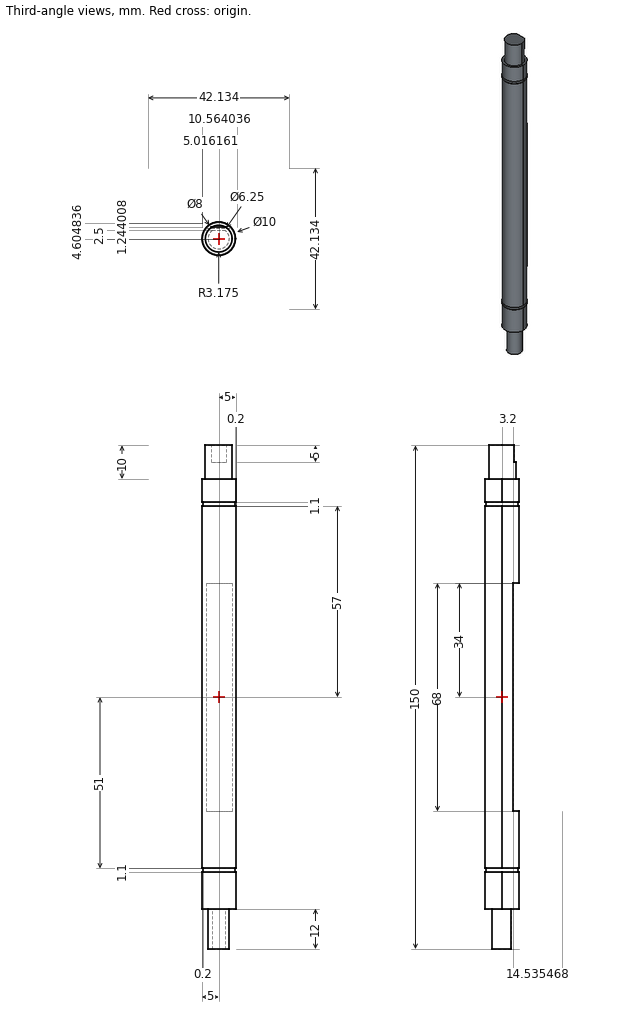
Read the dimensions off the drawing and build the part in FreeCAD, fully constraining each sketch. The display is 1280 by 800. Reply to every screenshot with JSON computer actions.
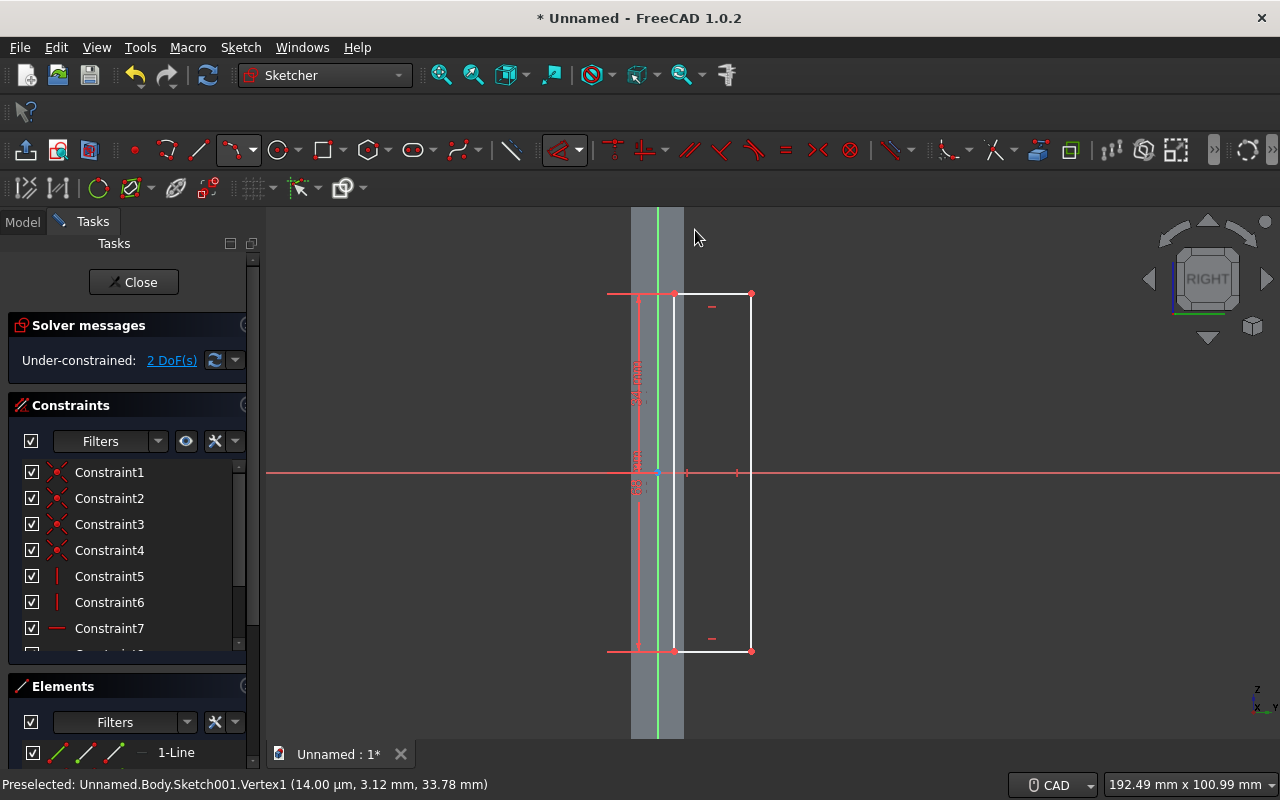
{"action": "scroll", "coordinate": [674, 294], "scroll_direction": "up", "scroll_amount": 5}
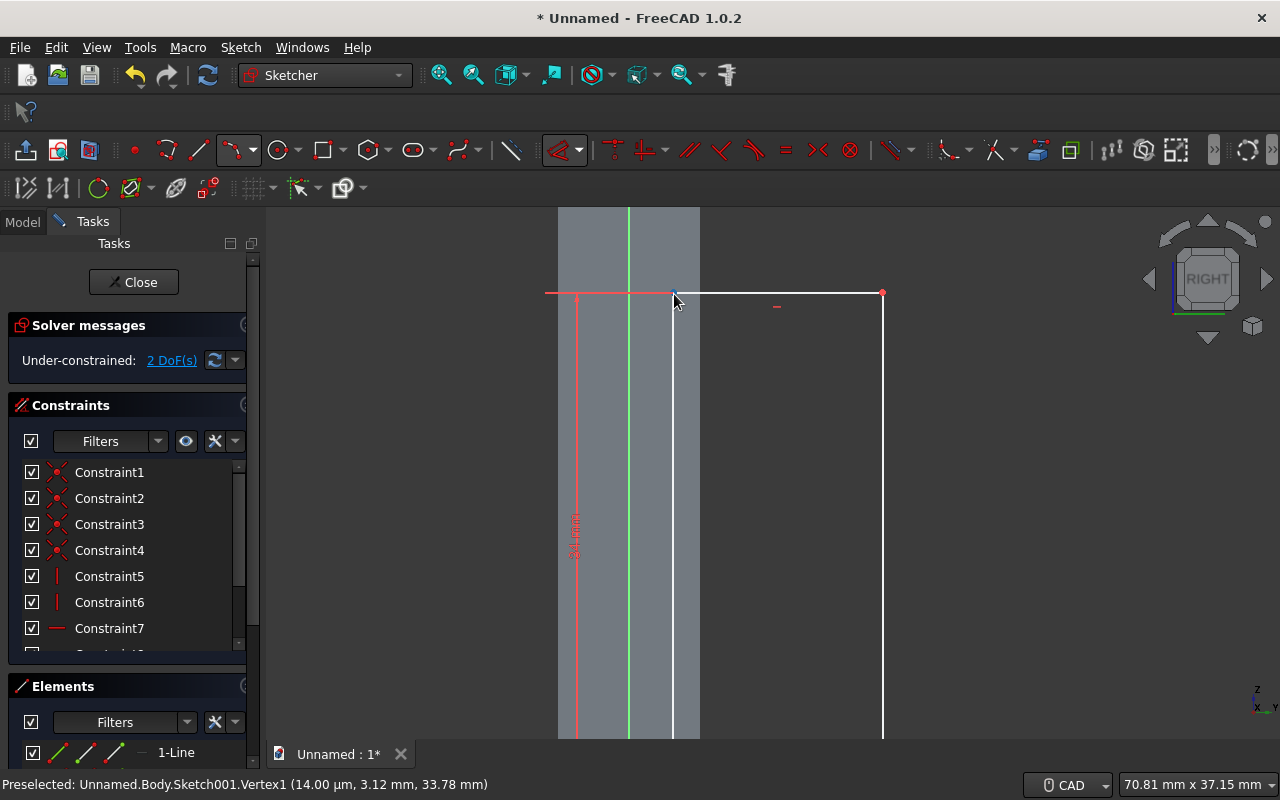
{"action": "left_click", "coordinate": [673, 293]}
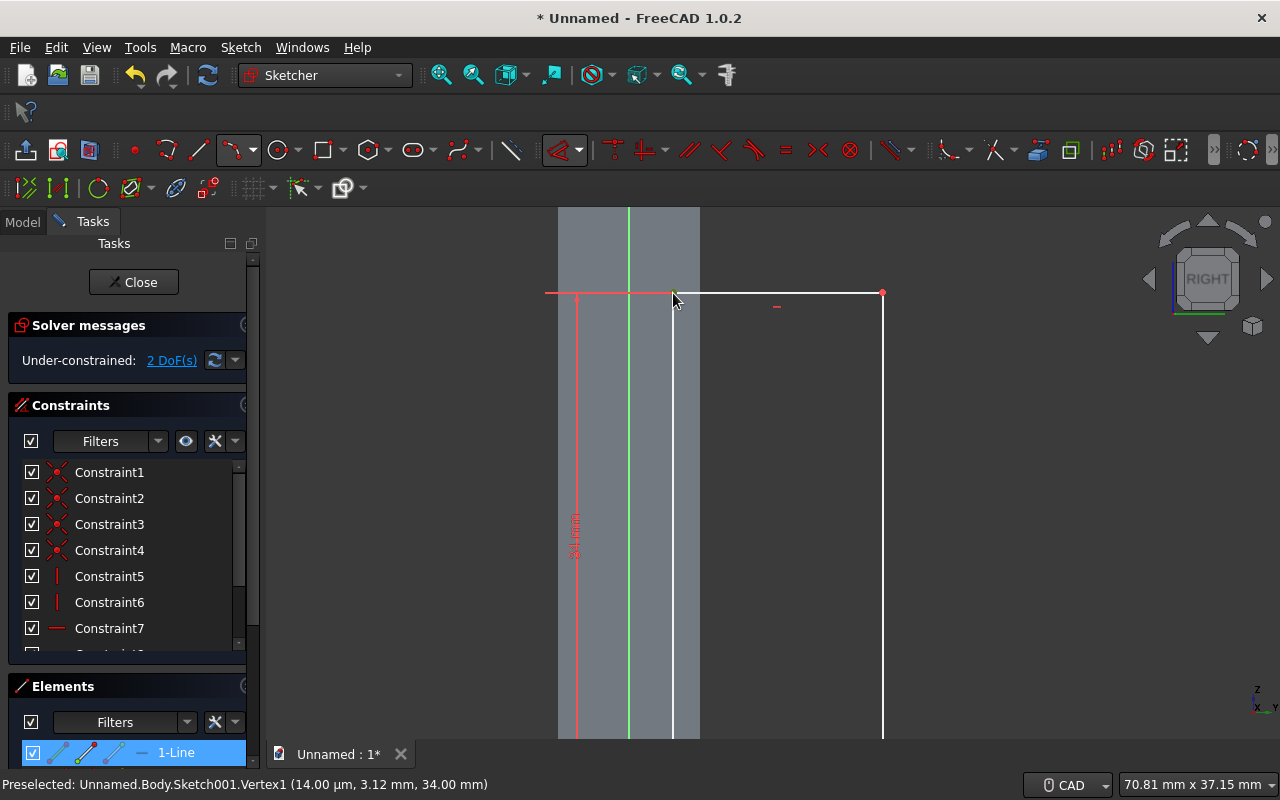
{"action": "left_click", "coordinate": [582, 150]}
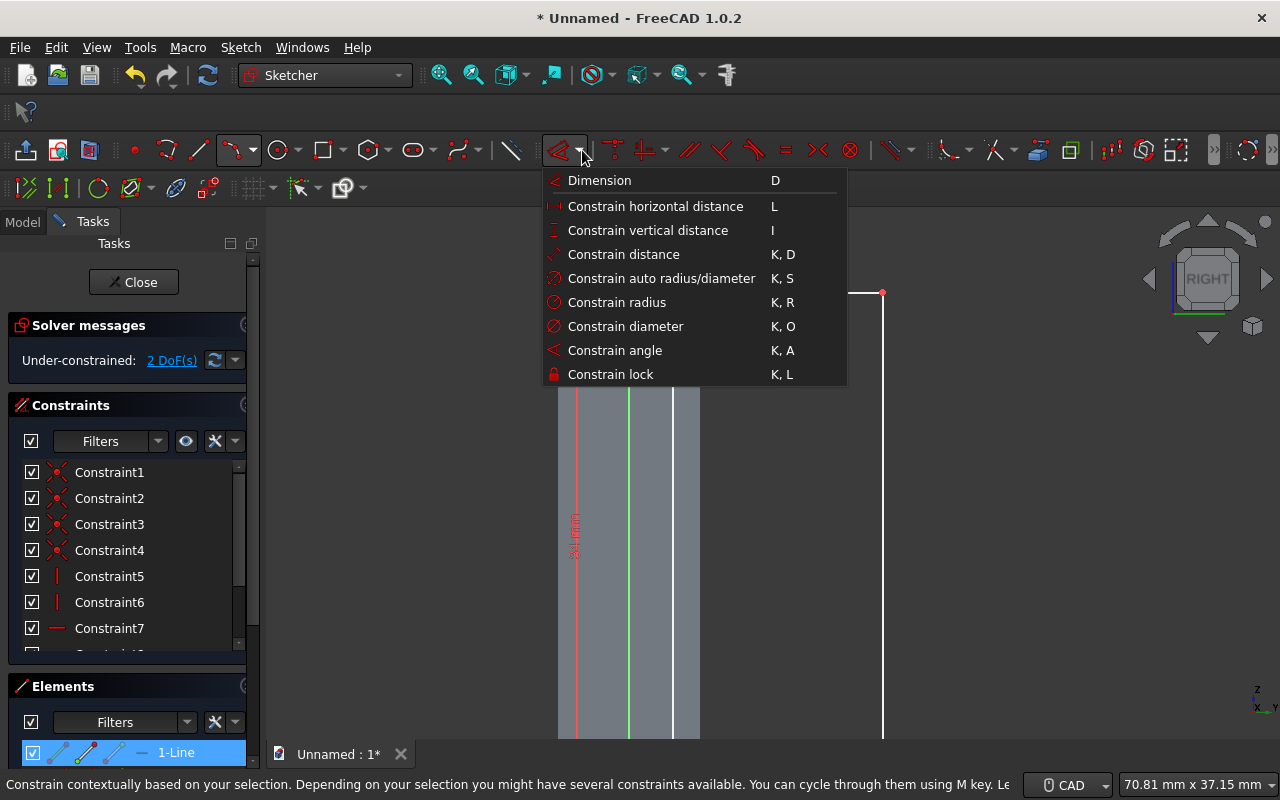
{"action": "left_click", "coordinate": [695, 206]}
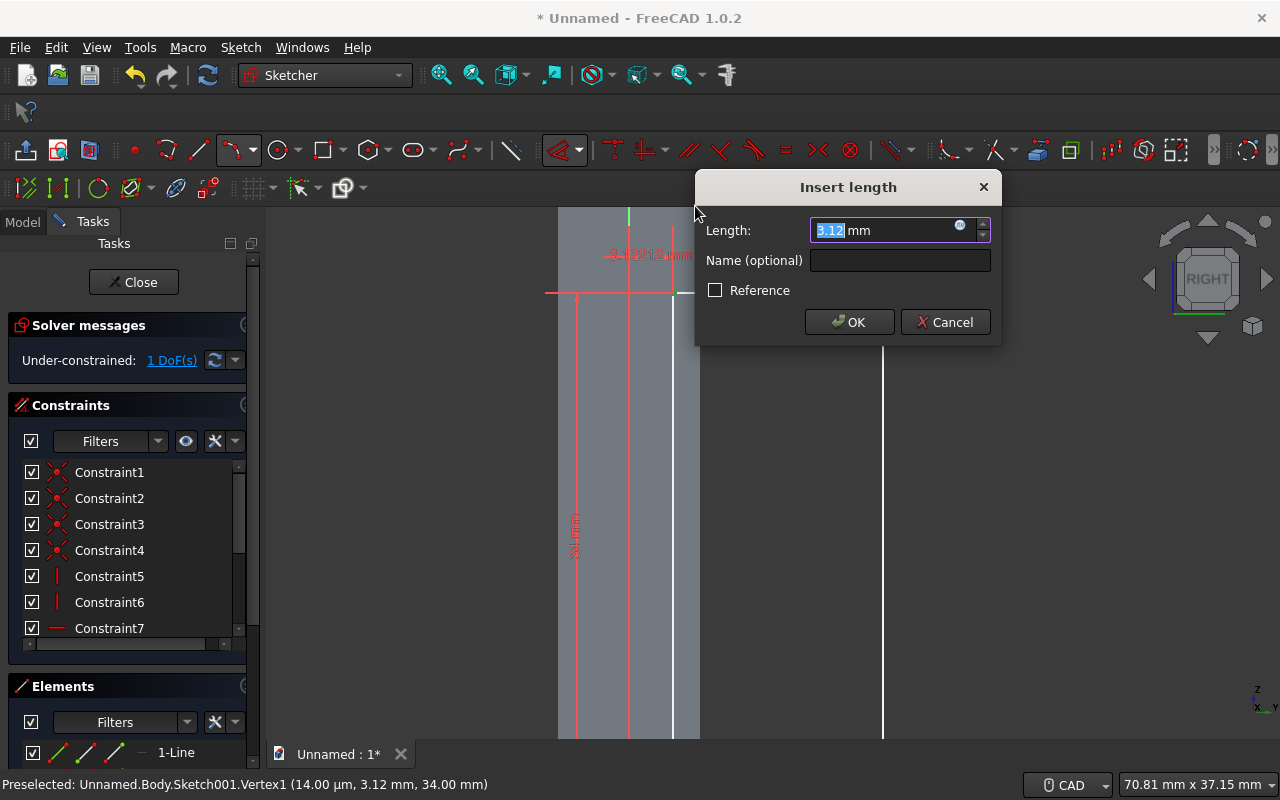
{"action": "type", "text": "3.2"}
{"action": "key", "text": "Return"}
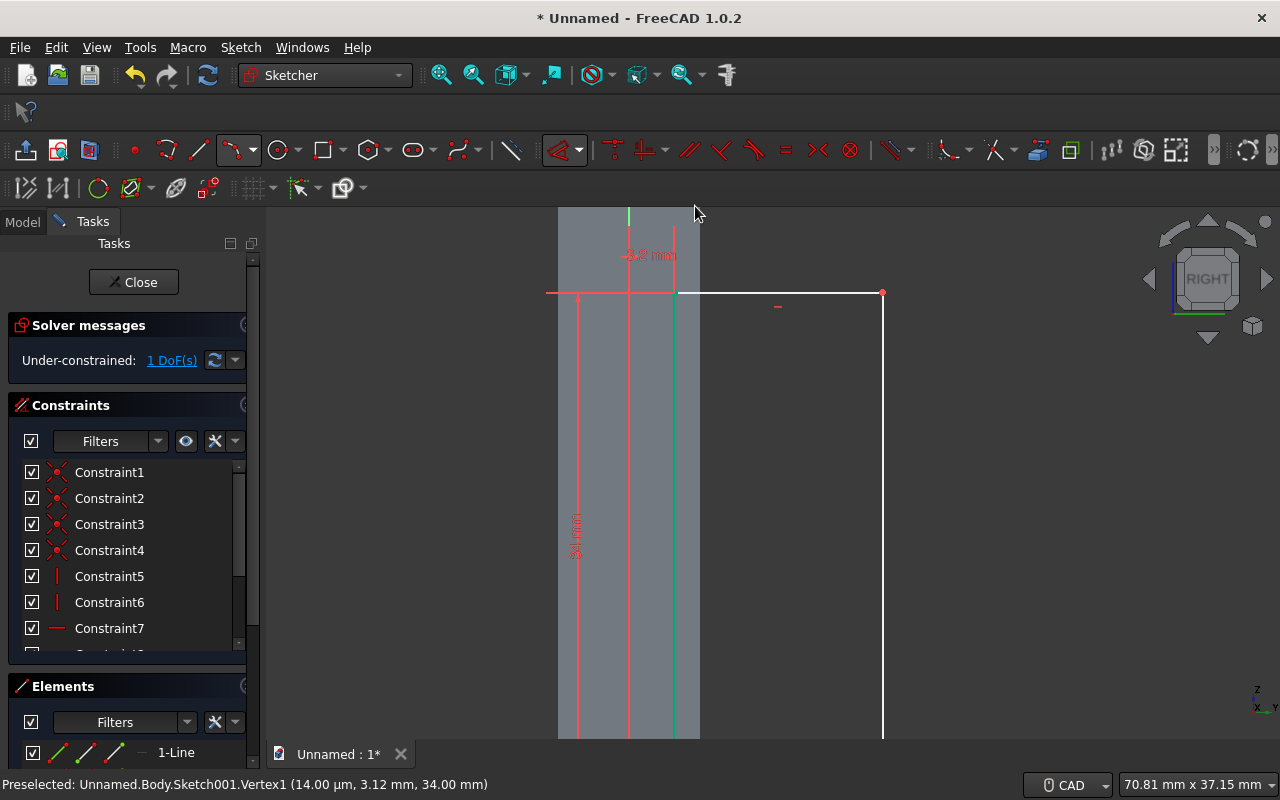
{"action": "scroll", "coordinate": [675, 295], "scroll_direction": "down", "scroll_amount": 5}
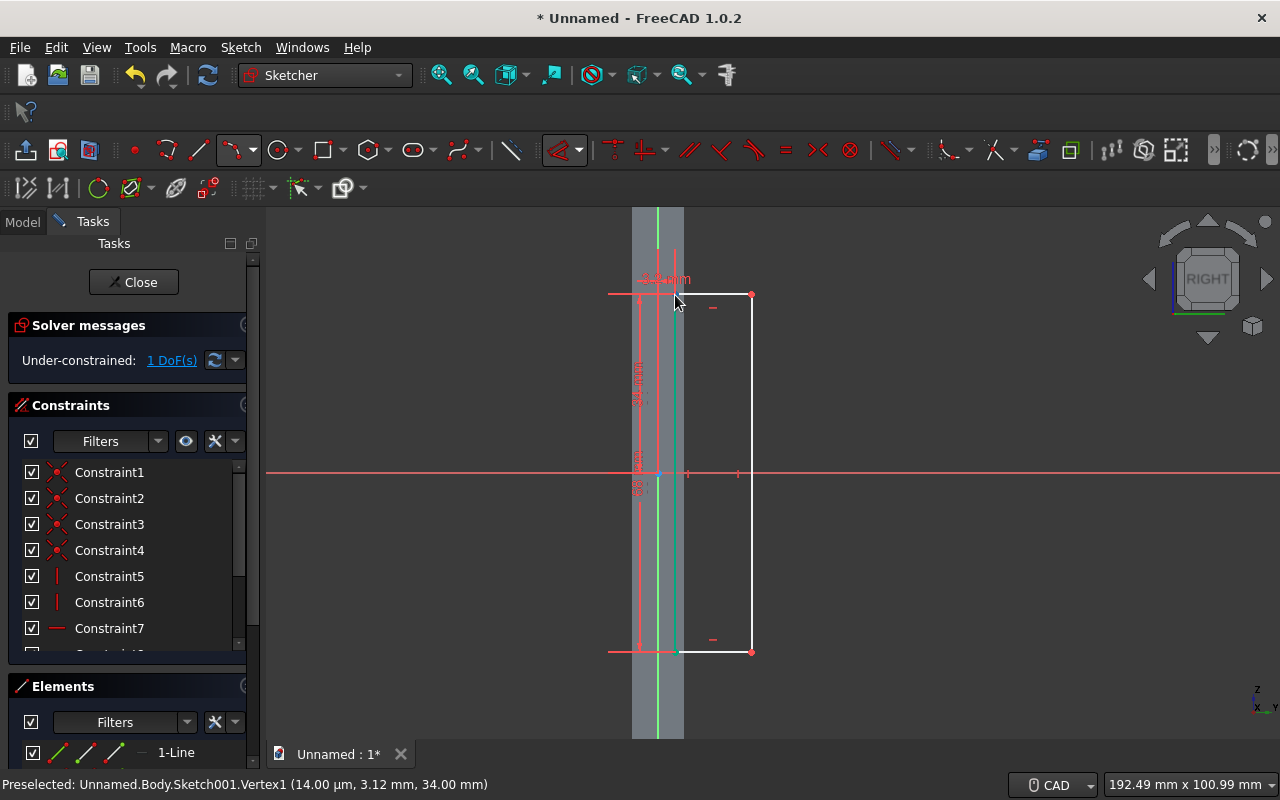
{"action": "left_click", "coordinate": [698, 652]}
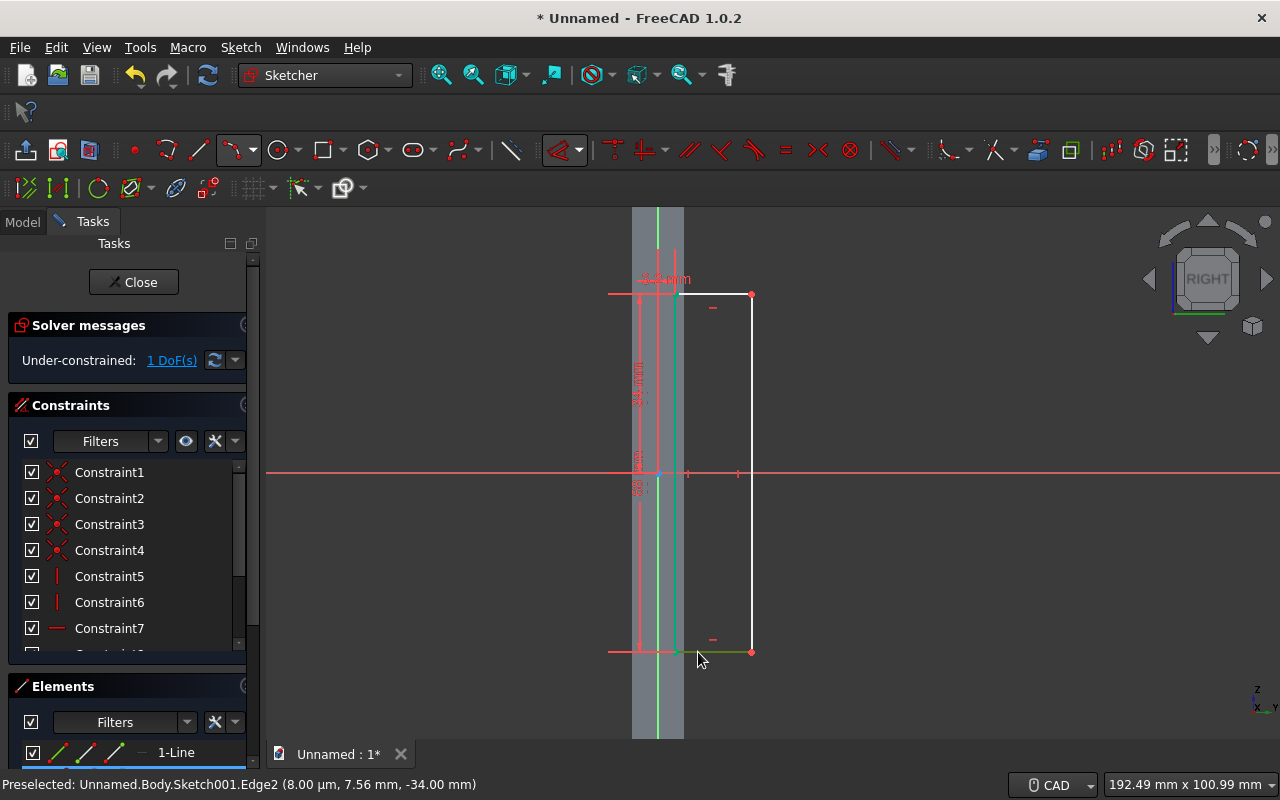
{"action": "key", "text": "l"}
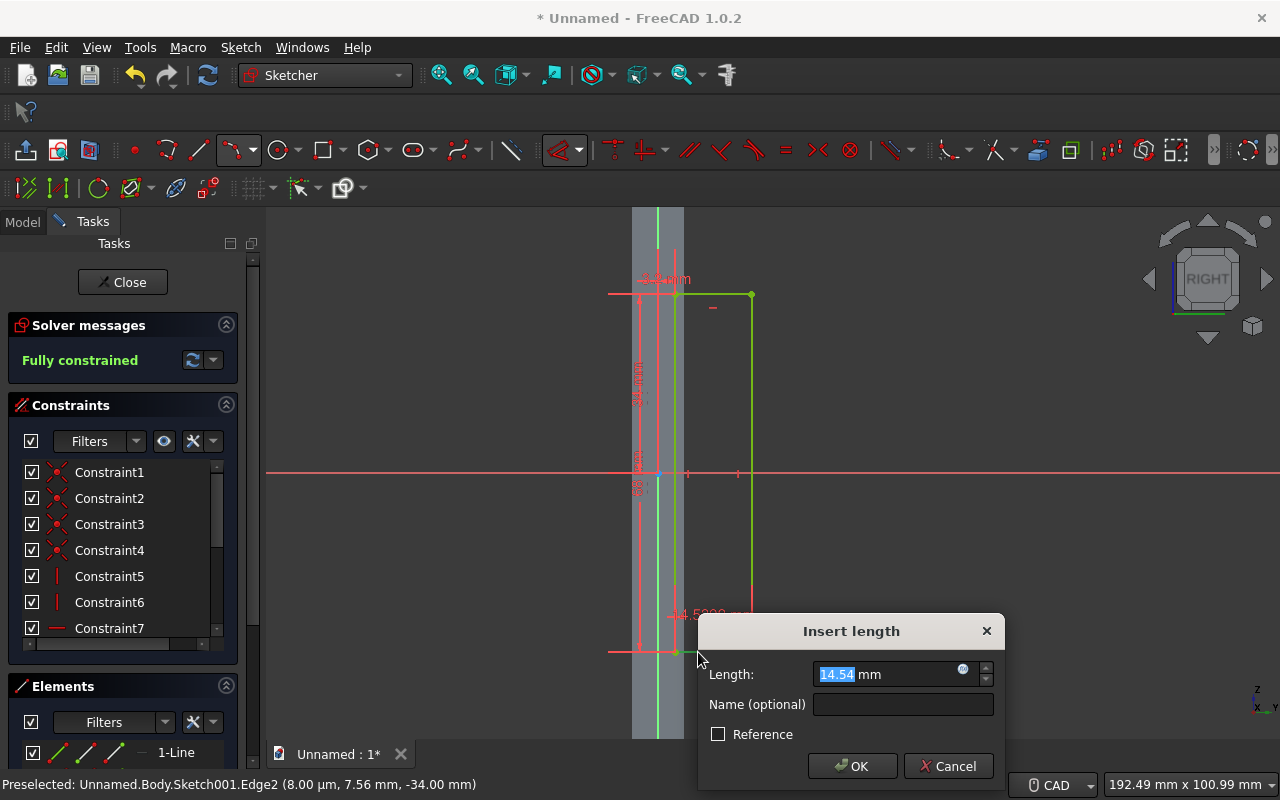
{"action": "type", "text": "14.535468"}
{"action": "key", "text": "Return"}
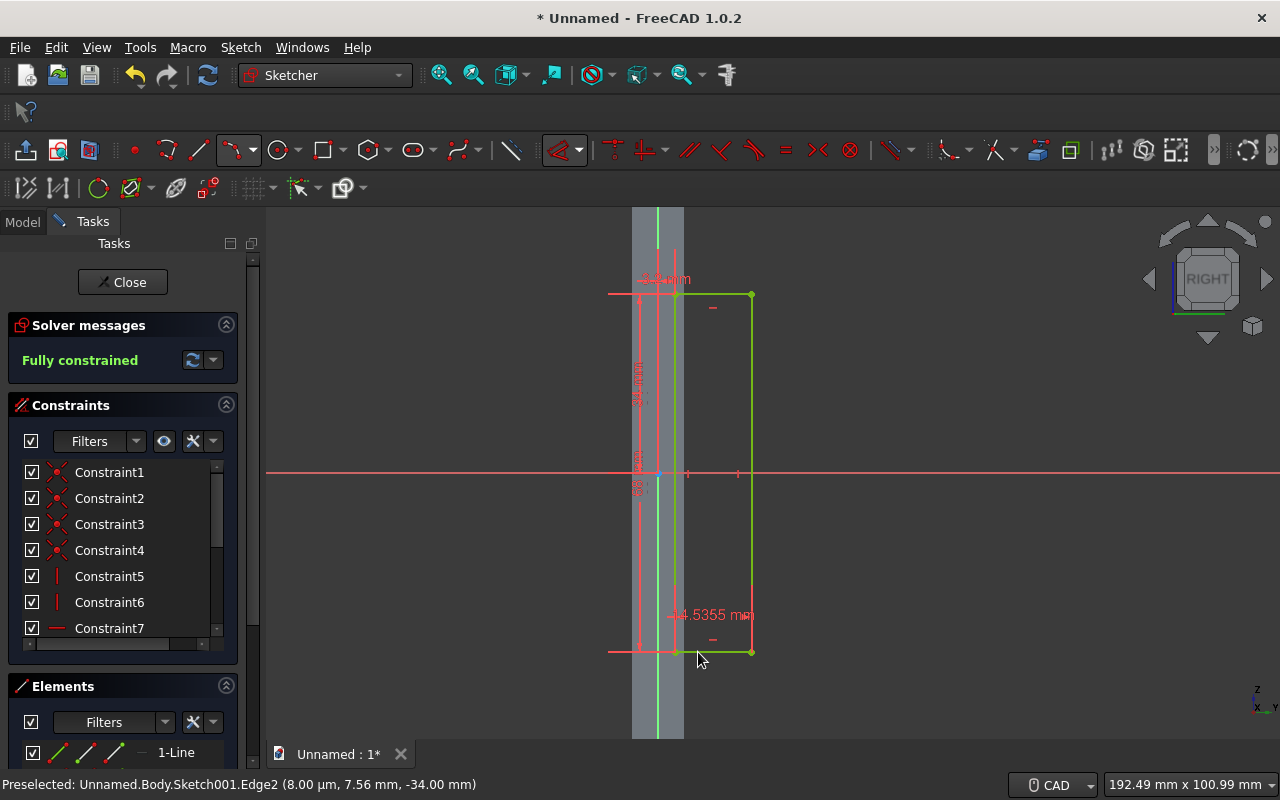
{"action": "left_click", "coordinate": [123, 282]}